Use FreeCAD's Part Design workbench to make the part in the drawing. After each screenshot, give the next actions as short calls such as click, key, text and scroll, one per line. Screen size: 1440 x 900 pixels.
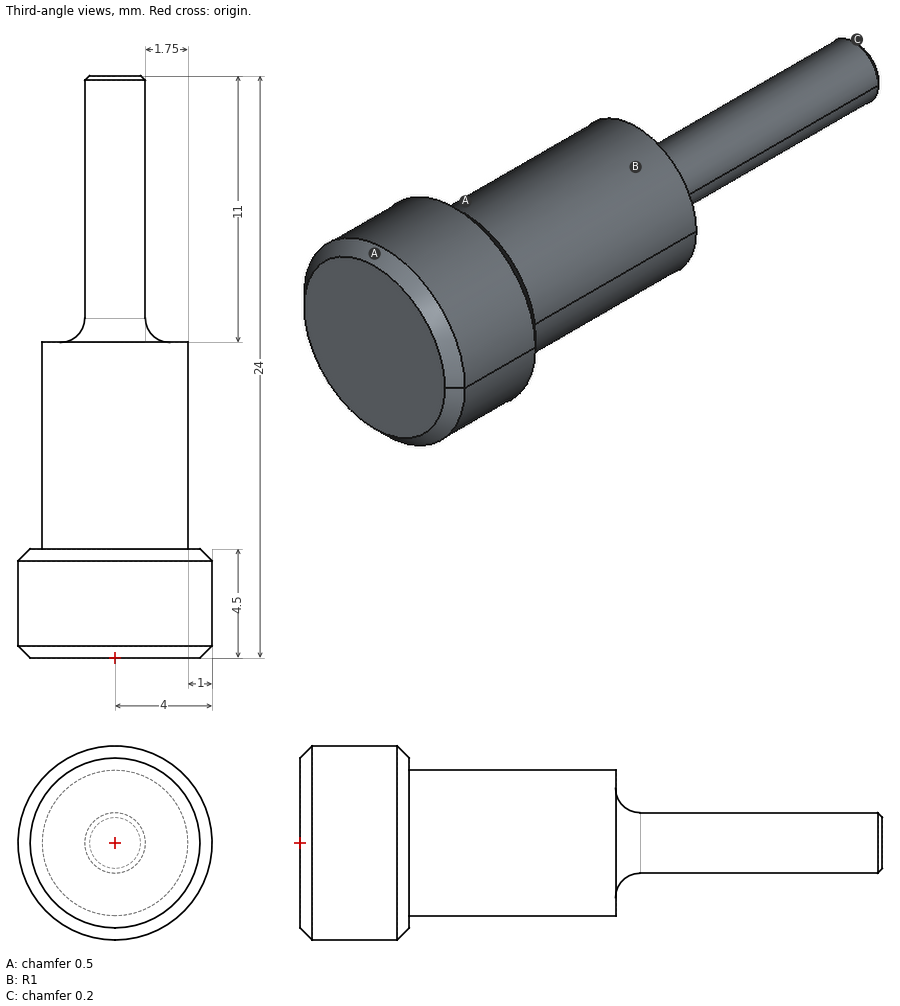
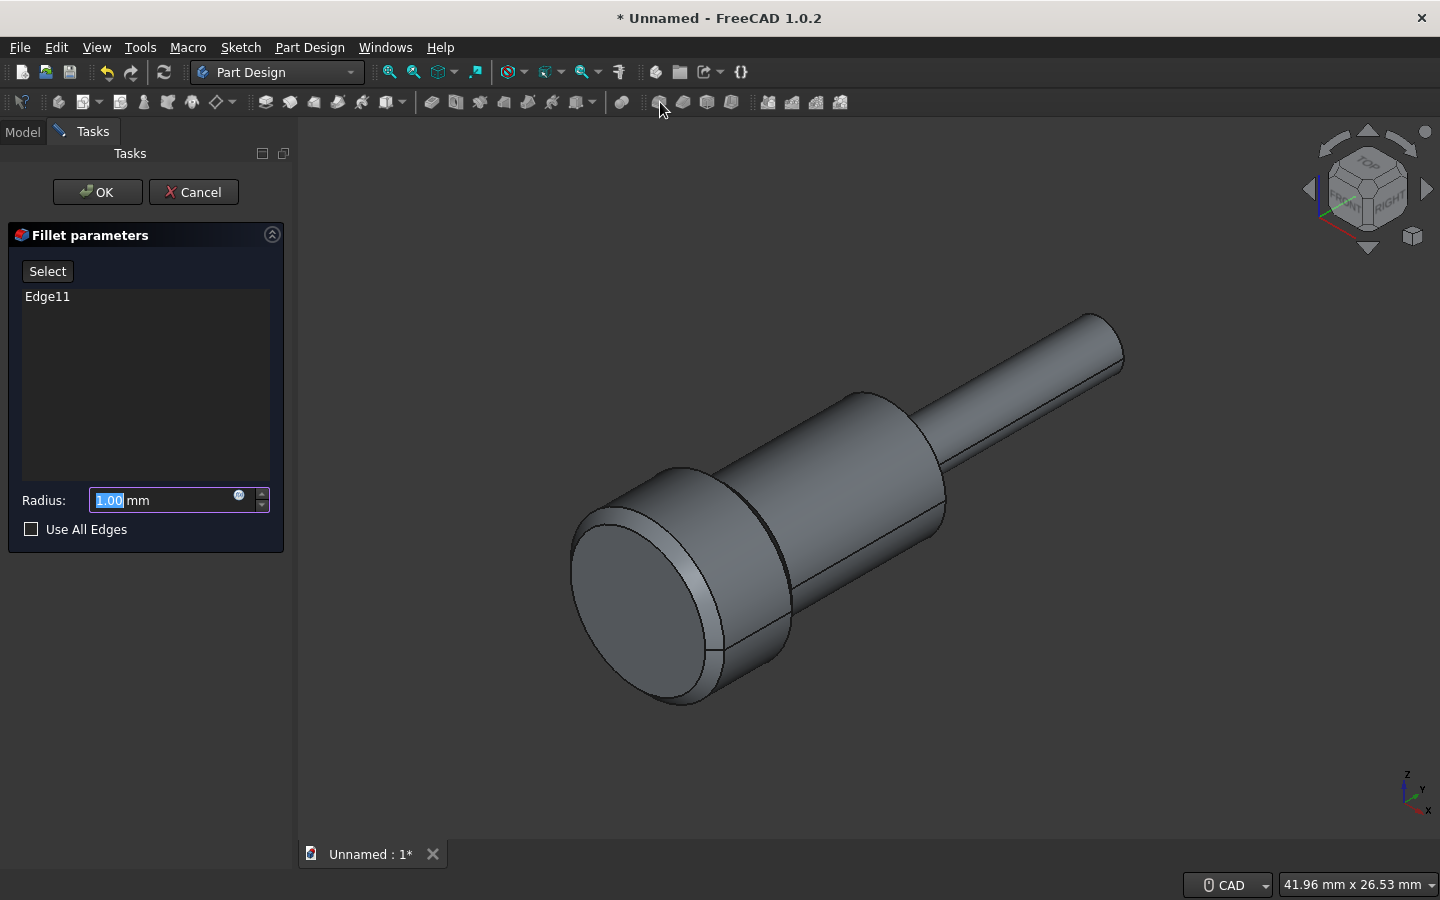
text(1)
key(Tab)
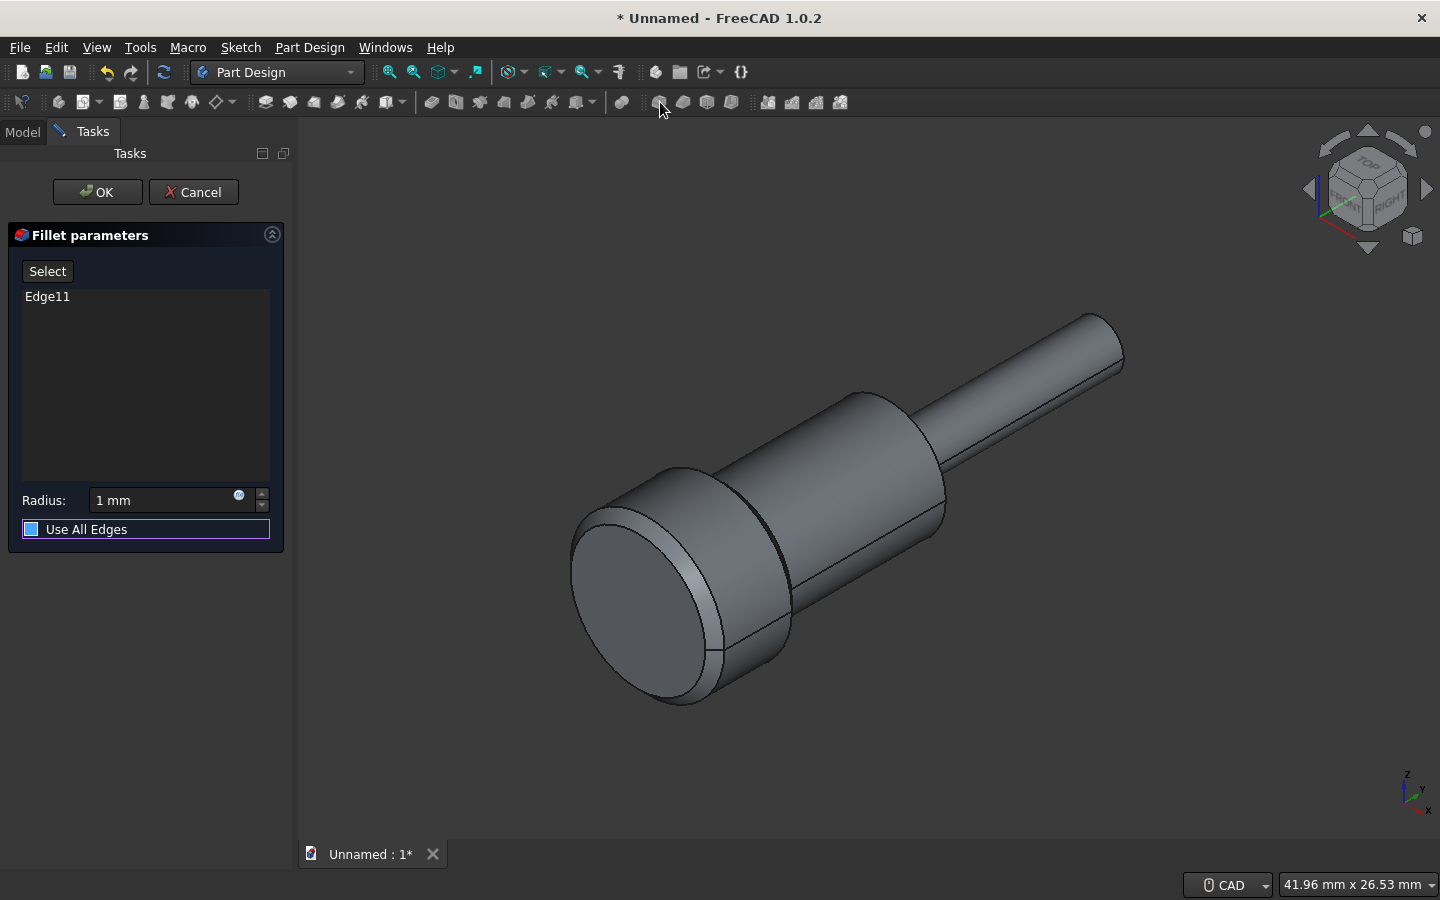
click(98, 192)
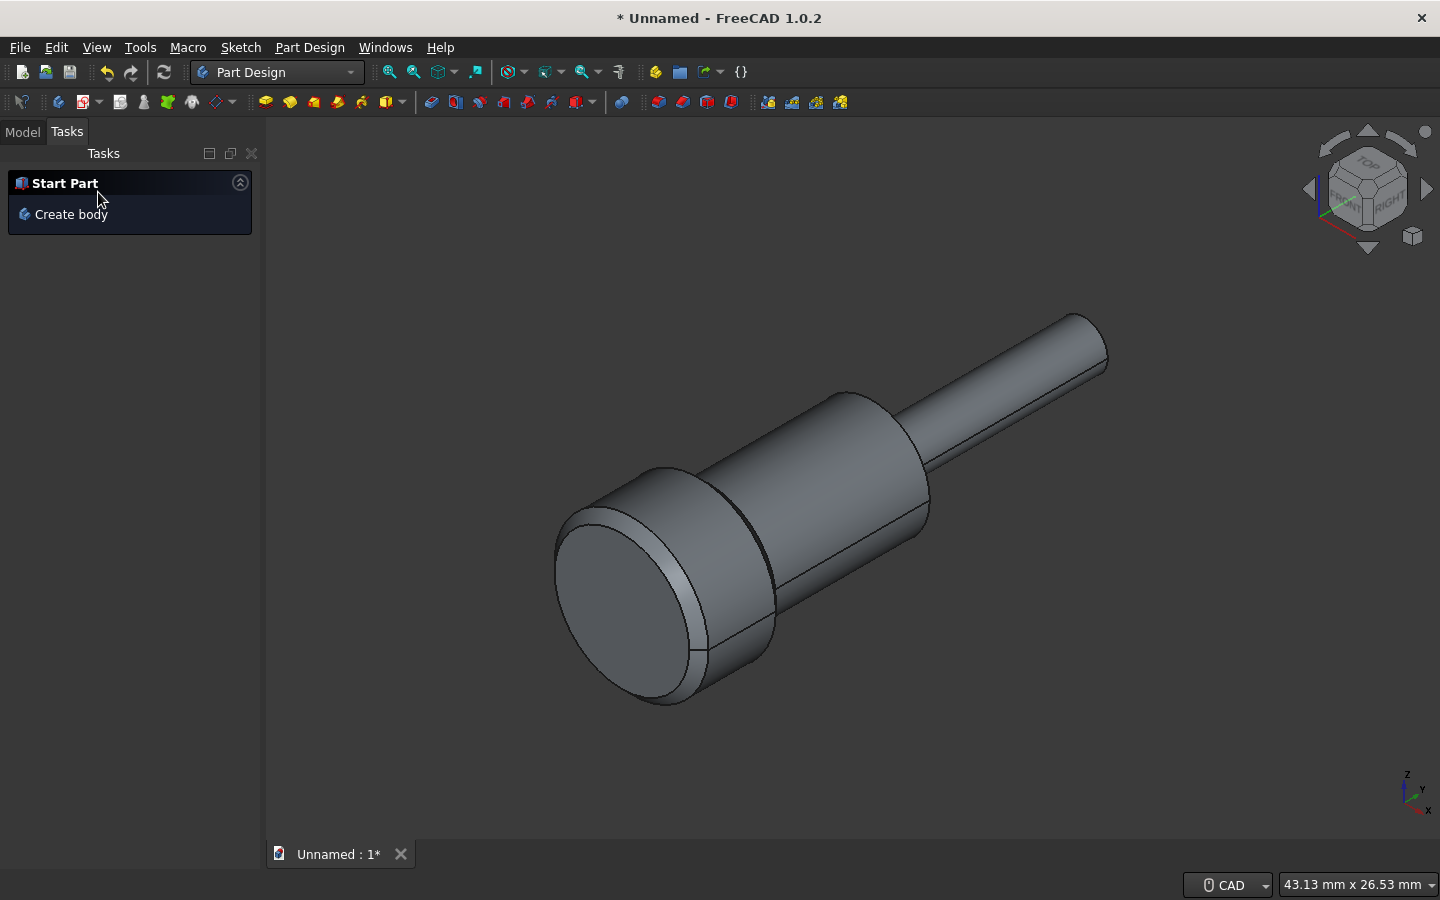
key(2)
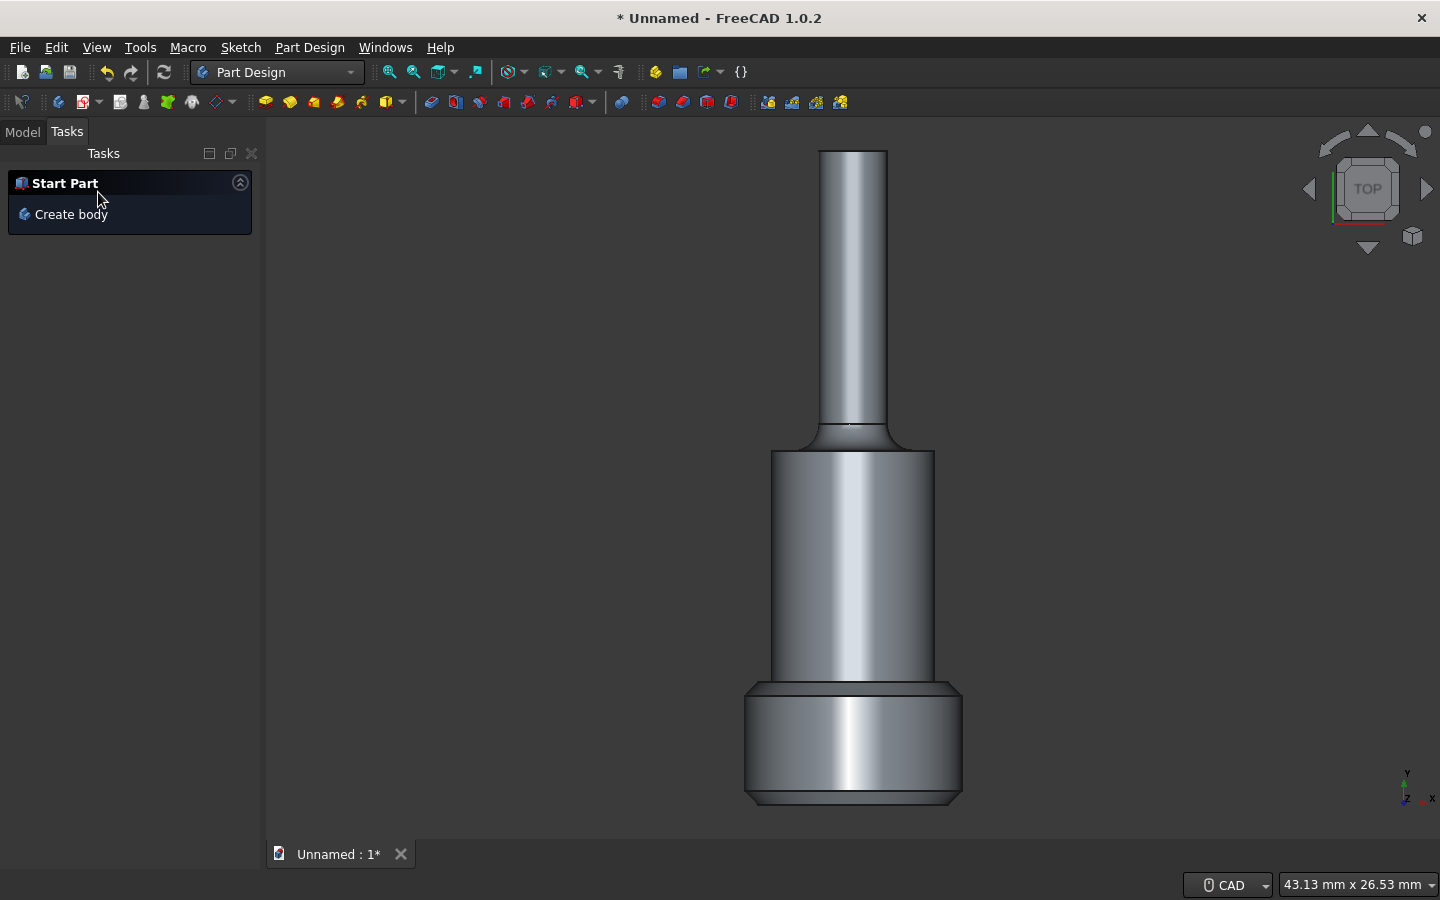
click(825, 150)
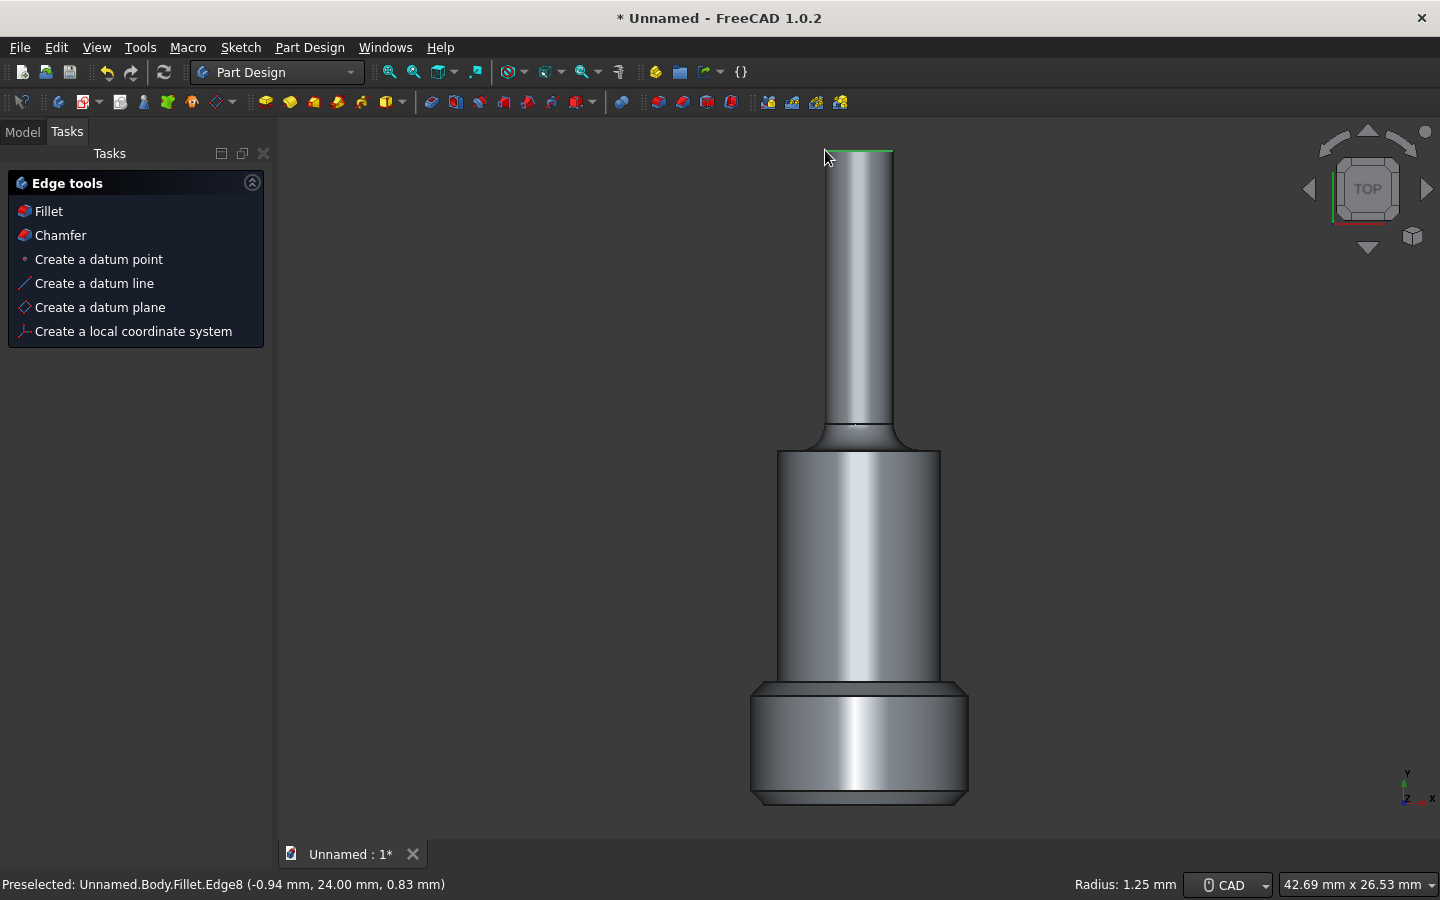
click(684, 102)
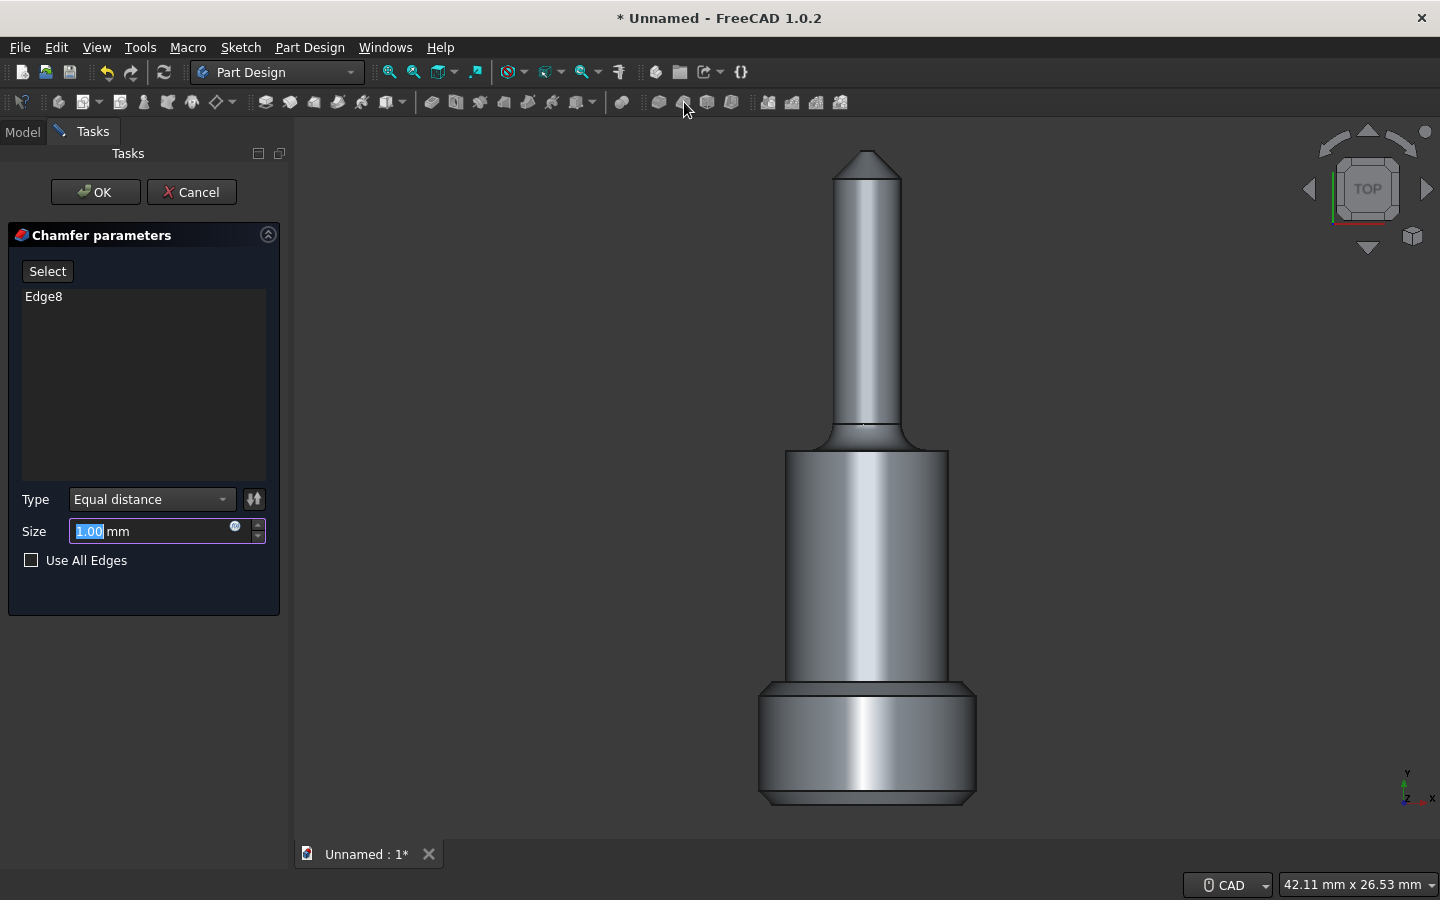
text(0.2)
key(Tab)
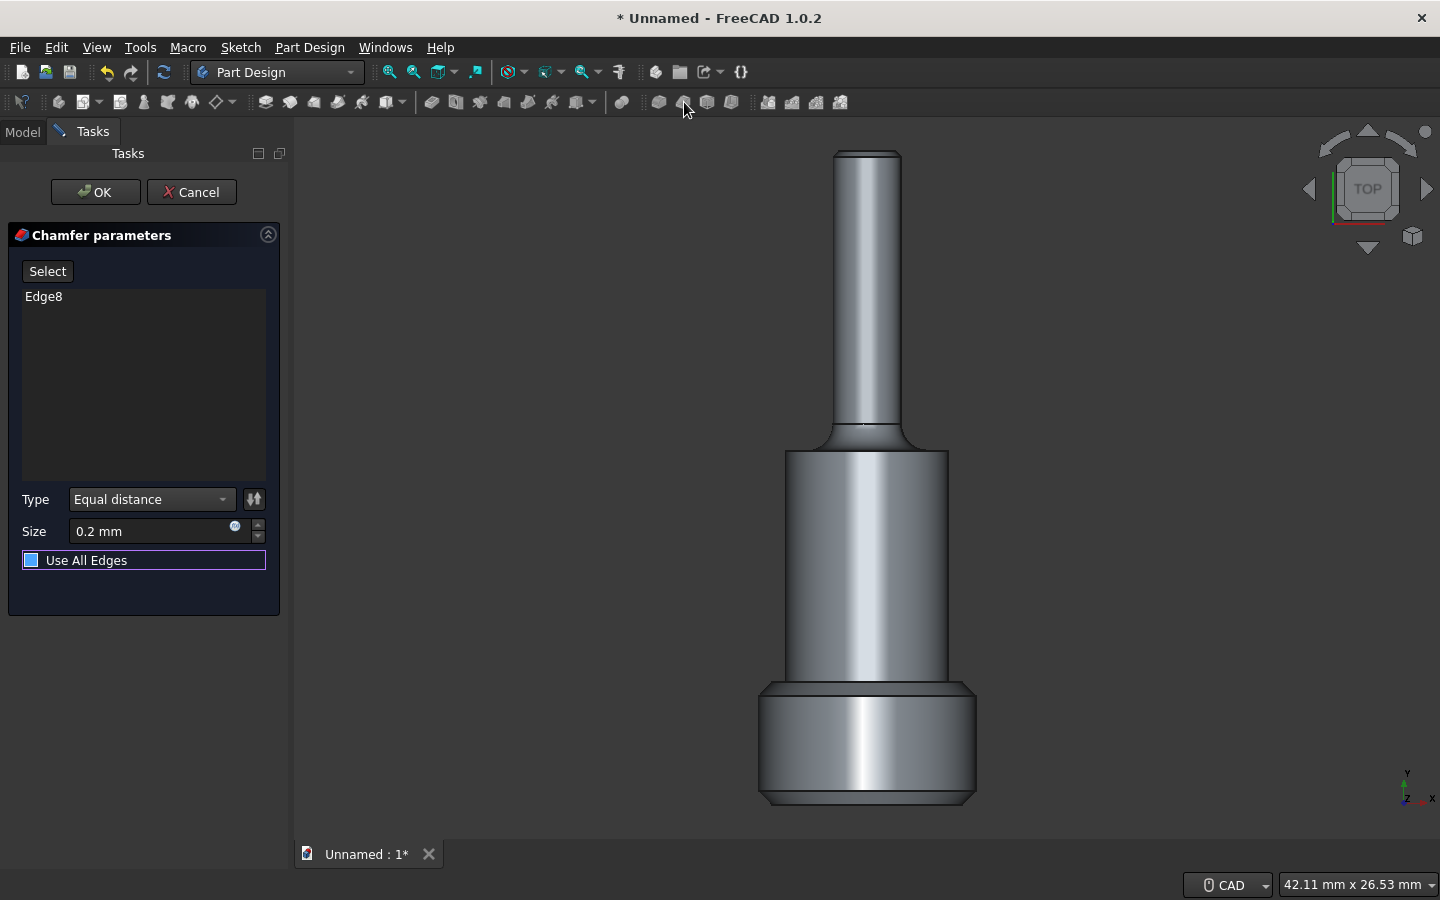
click(96, 192)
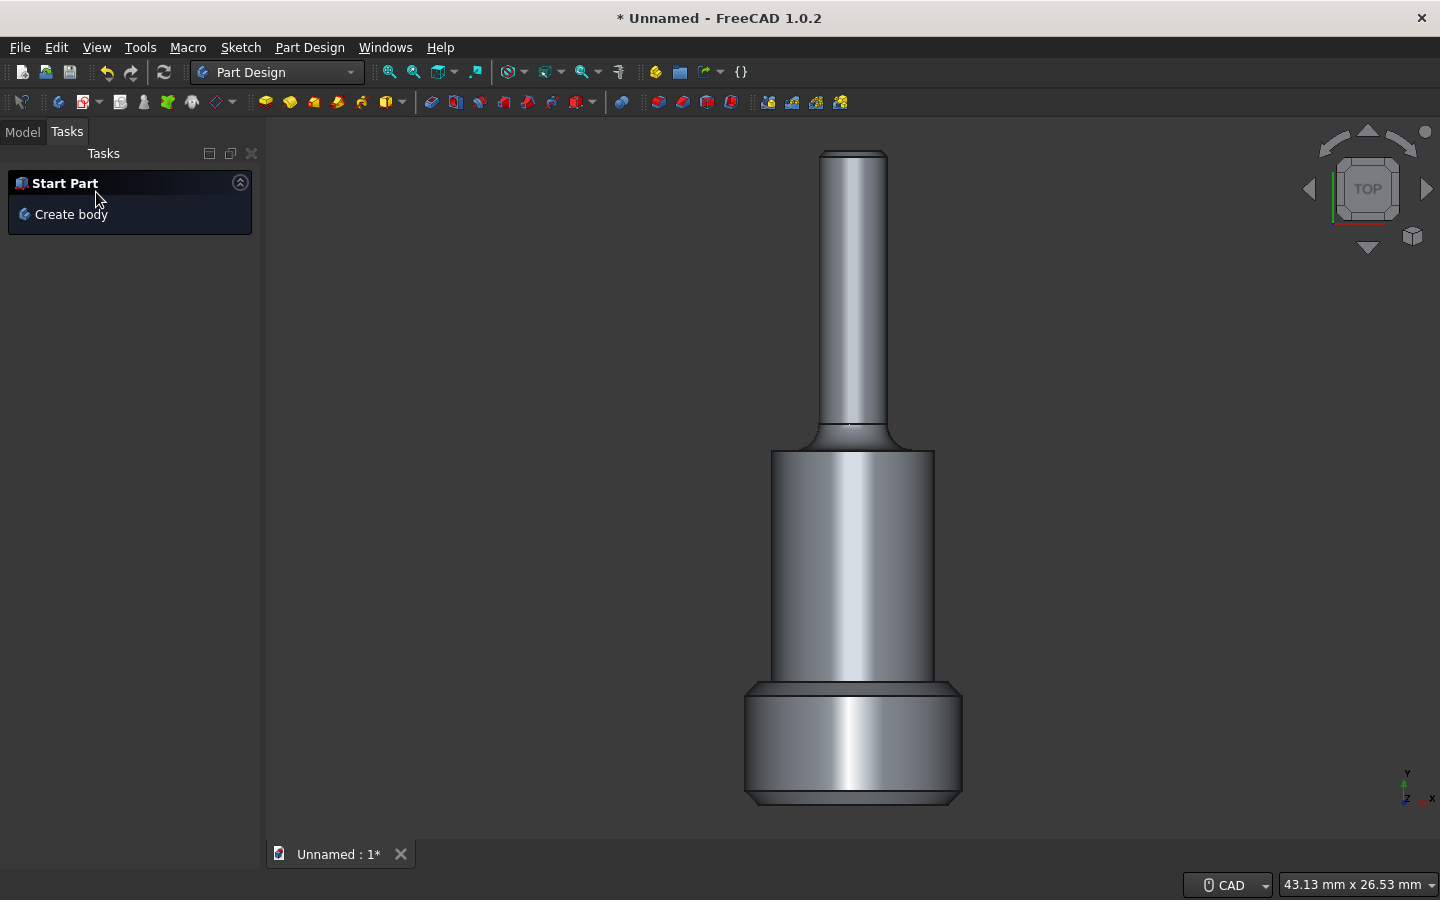
key(0)